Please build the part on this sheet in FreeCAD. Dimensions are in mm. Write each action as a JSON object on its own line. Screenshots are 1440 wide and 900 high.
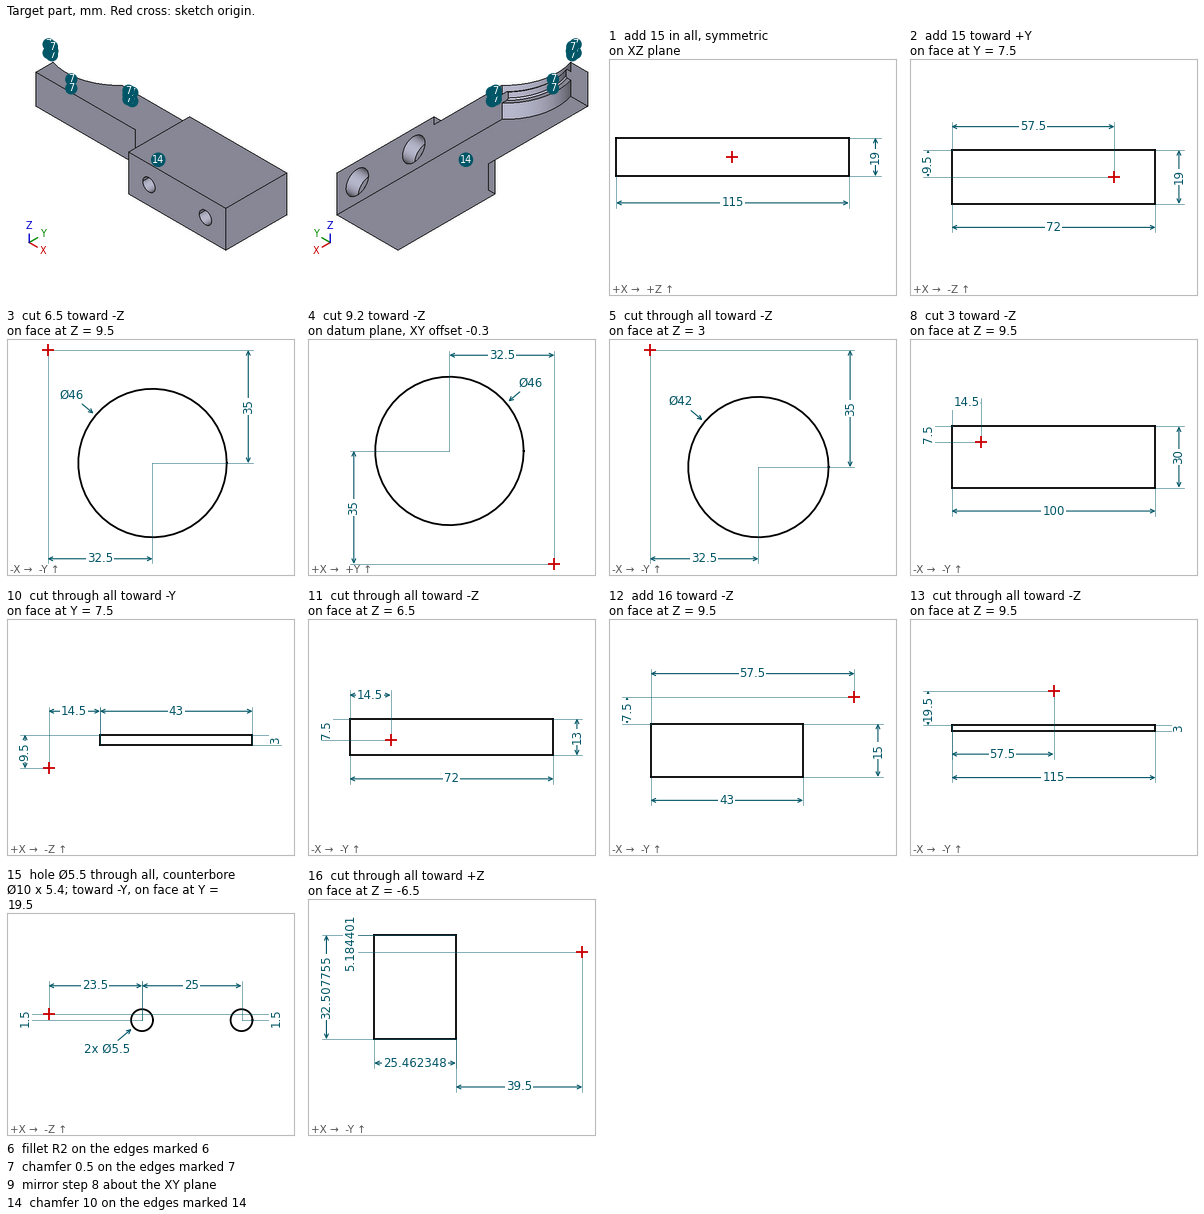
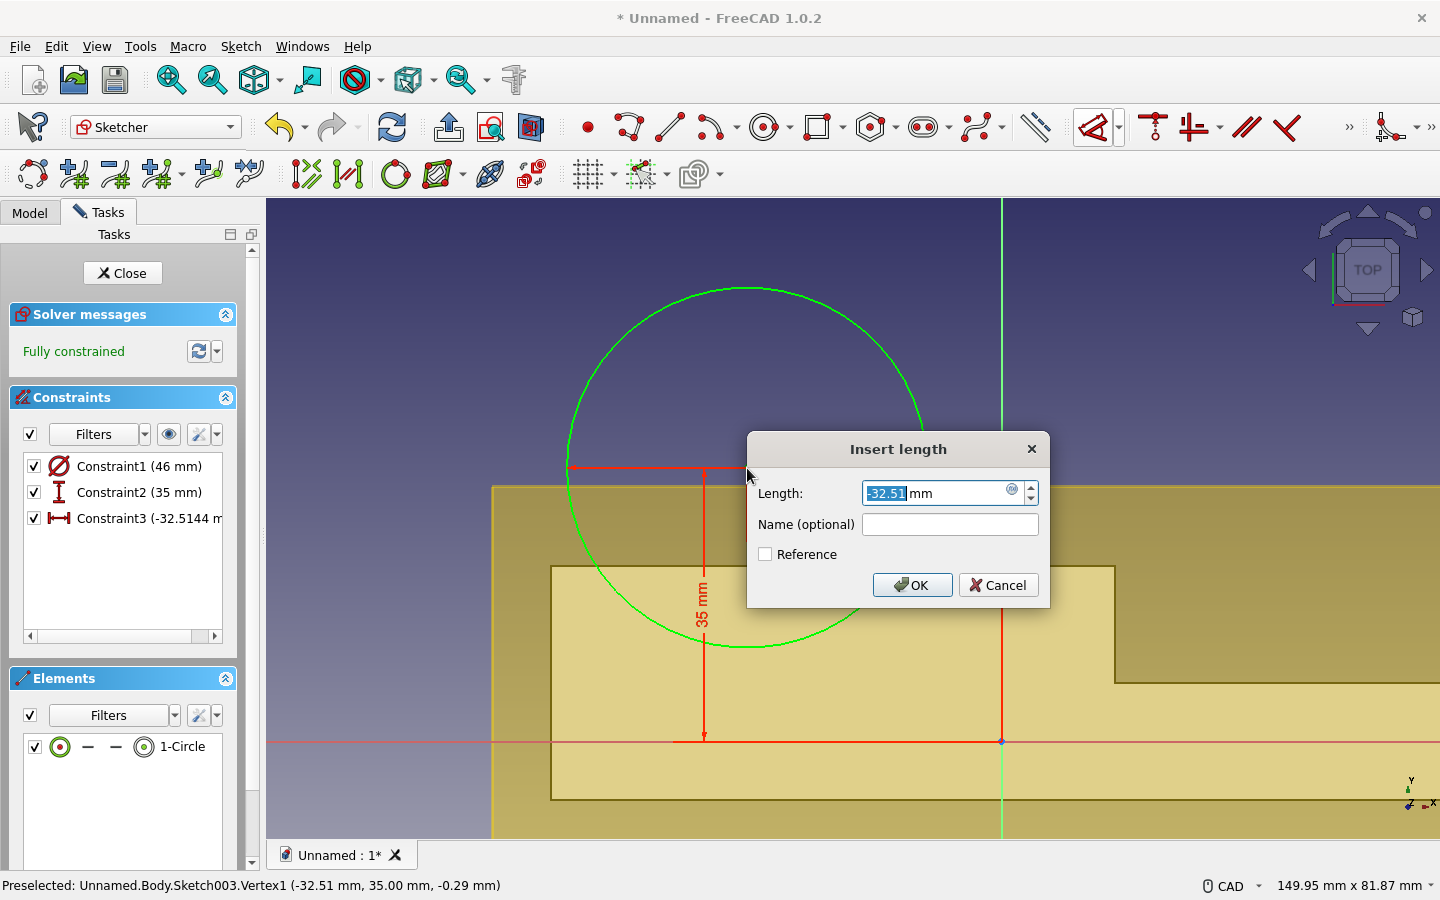
{"action": "type", "text": "-32.5"}
{"action": "key", "text": "Return"}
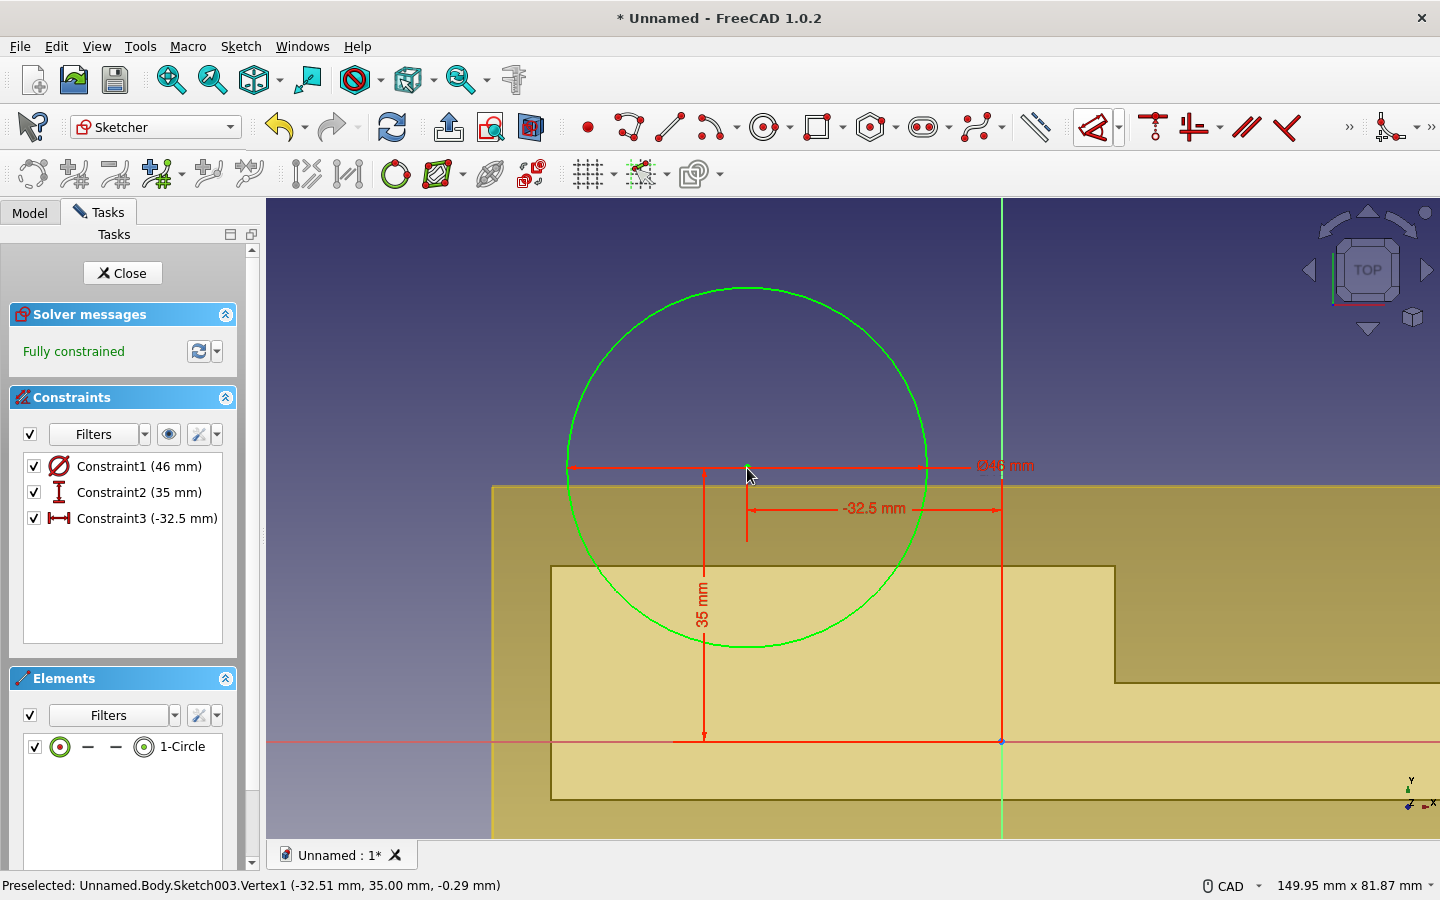
{"action": "left_click", "coordinate": [123, 273]}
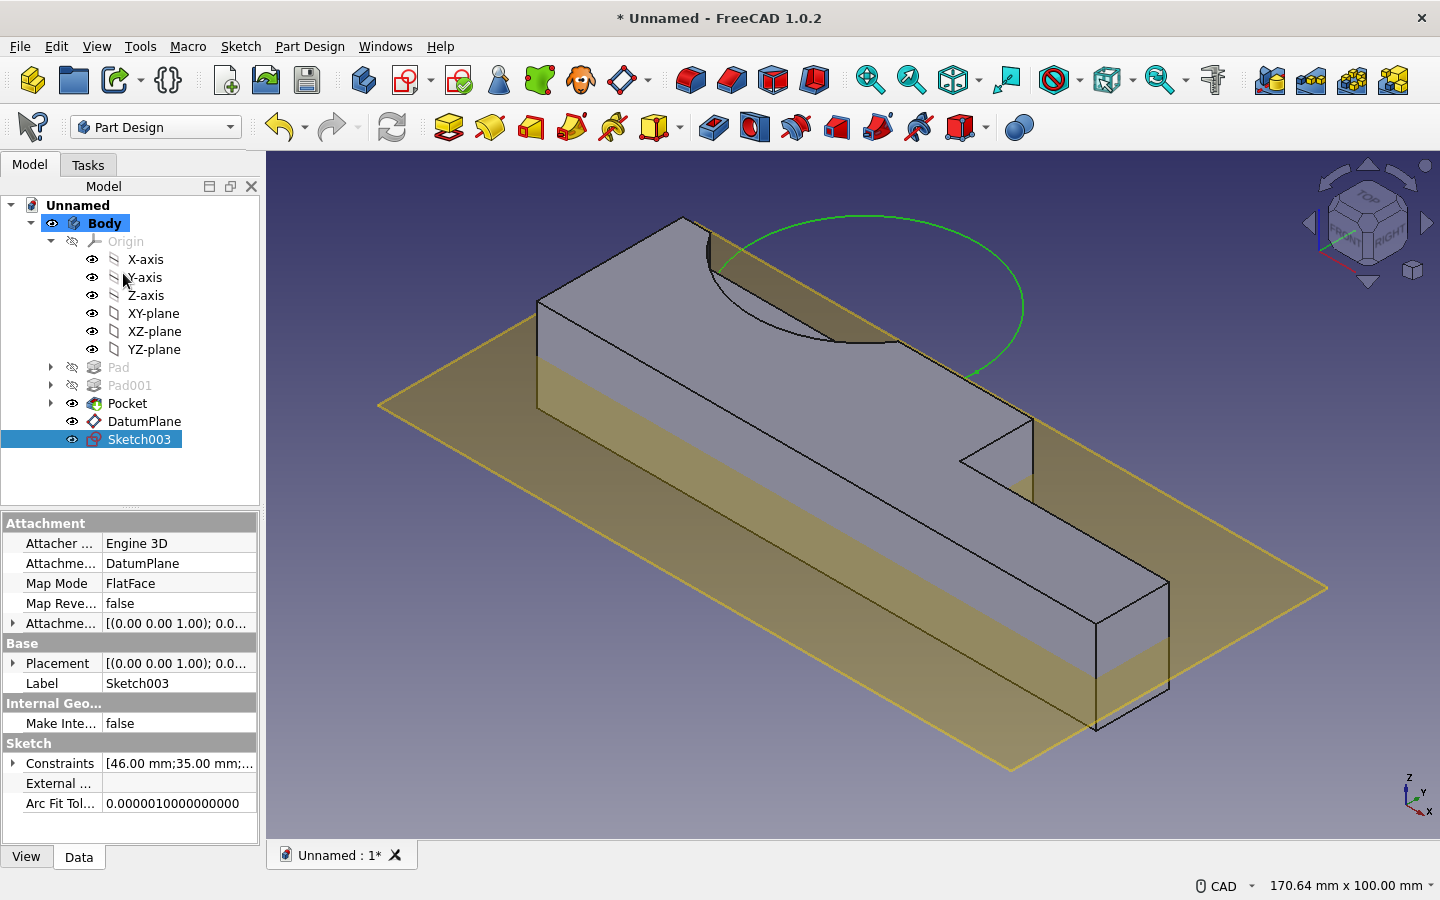
{"action": "left_click", "coordinate": [714, 128]}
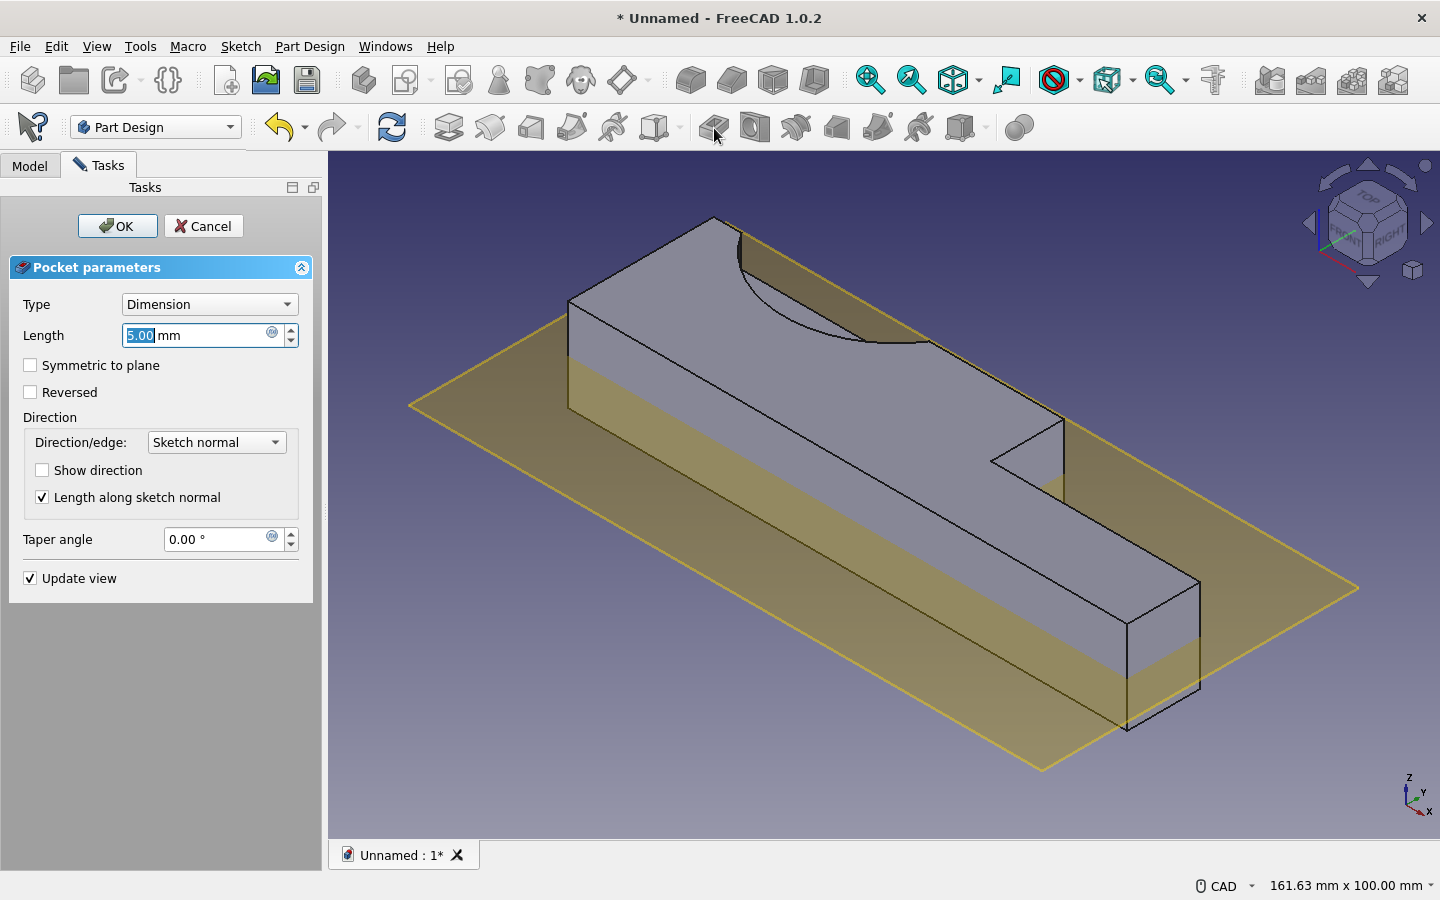
{"action": "type", "text": "9.2"}
{"action": "key", "text": "Tab"}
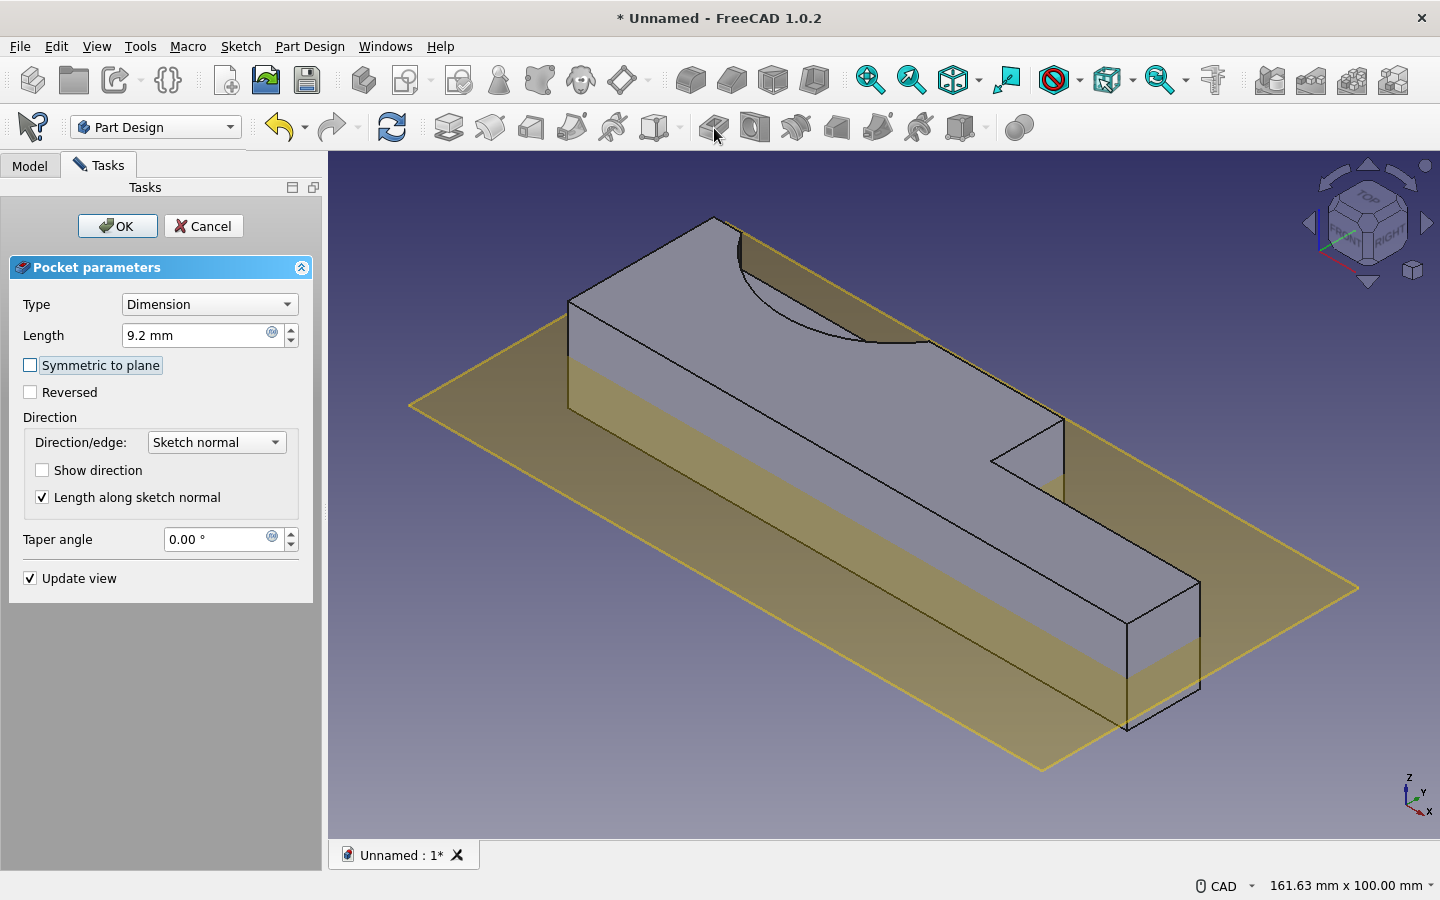
{"action": "left_click", "coordinate": [118, 226]}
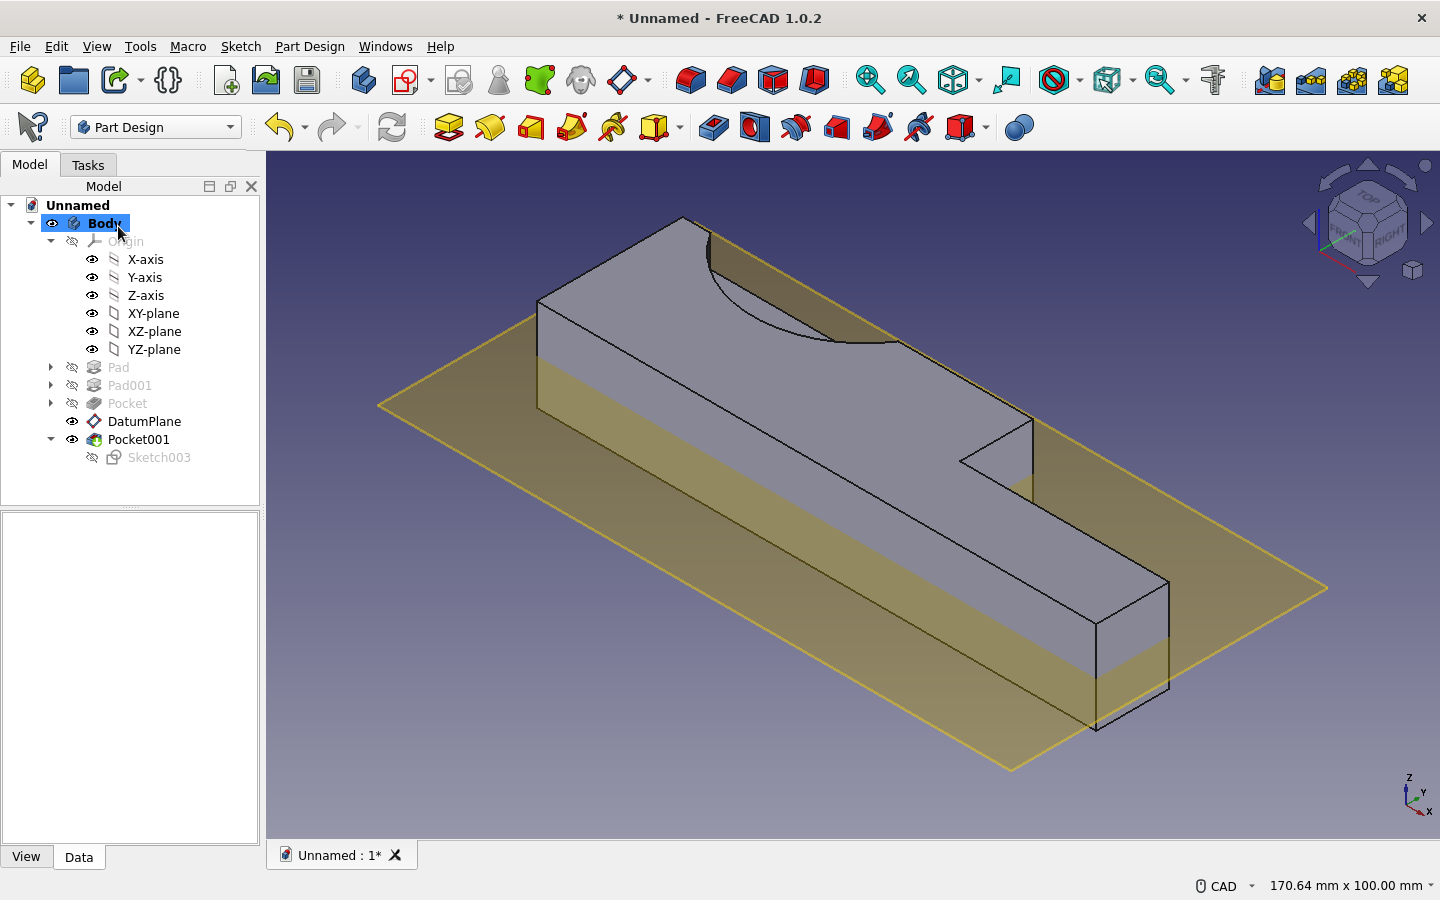
{"action": "left_click", "coordinate": [117, 421]}
{"action": "key", "text": "space"}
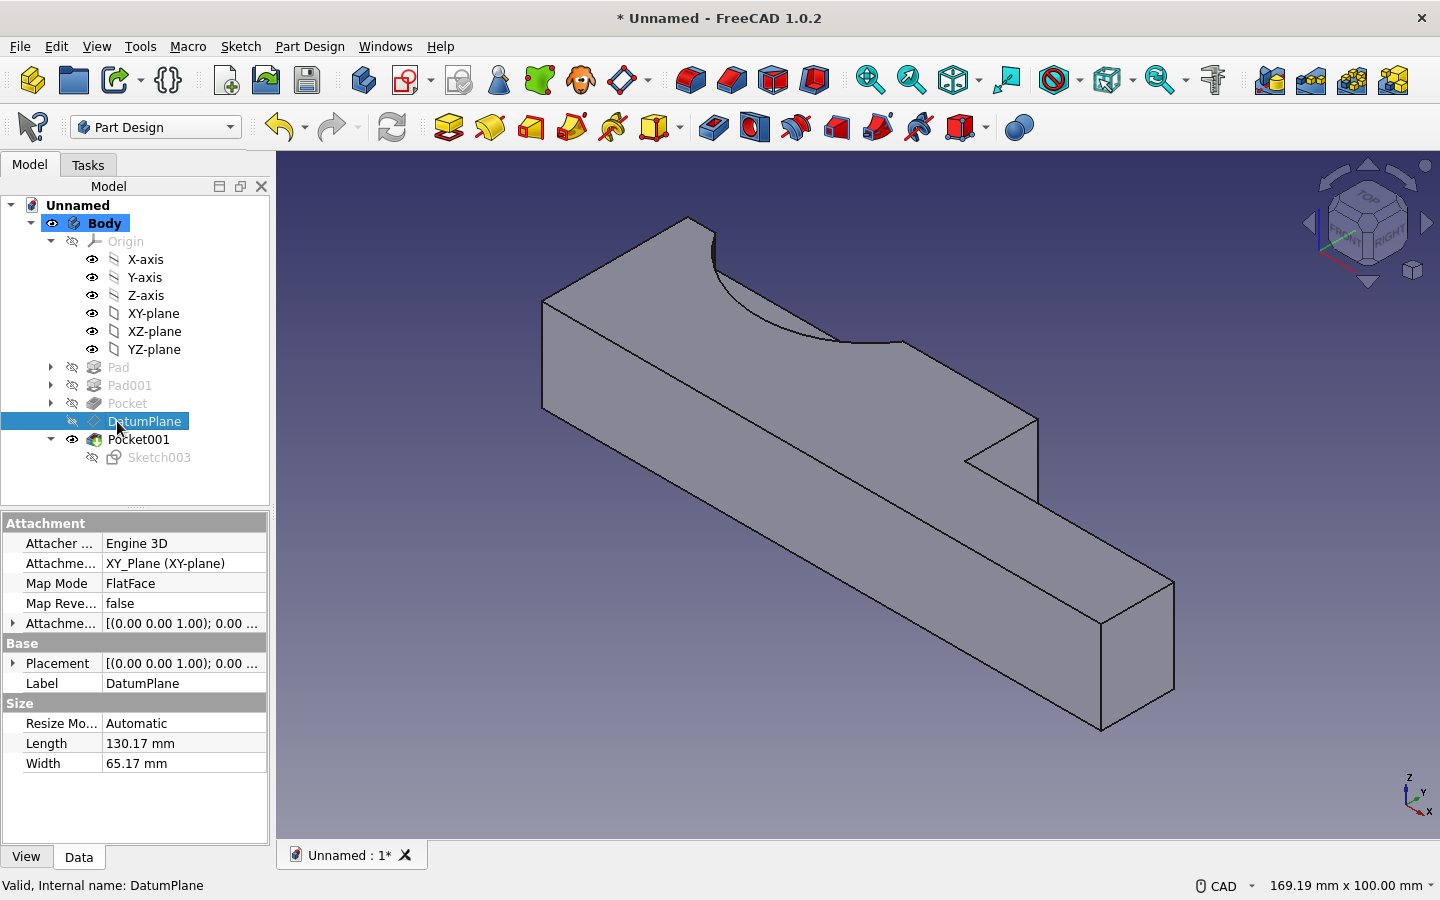
{"action": "key", "text": "2"}